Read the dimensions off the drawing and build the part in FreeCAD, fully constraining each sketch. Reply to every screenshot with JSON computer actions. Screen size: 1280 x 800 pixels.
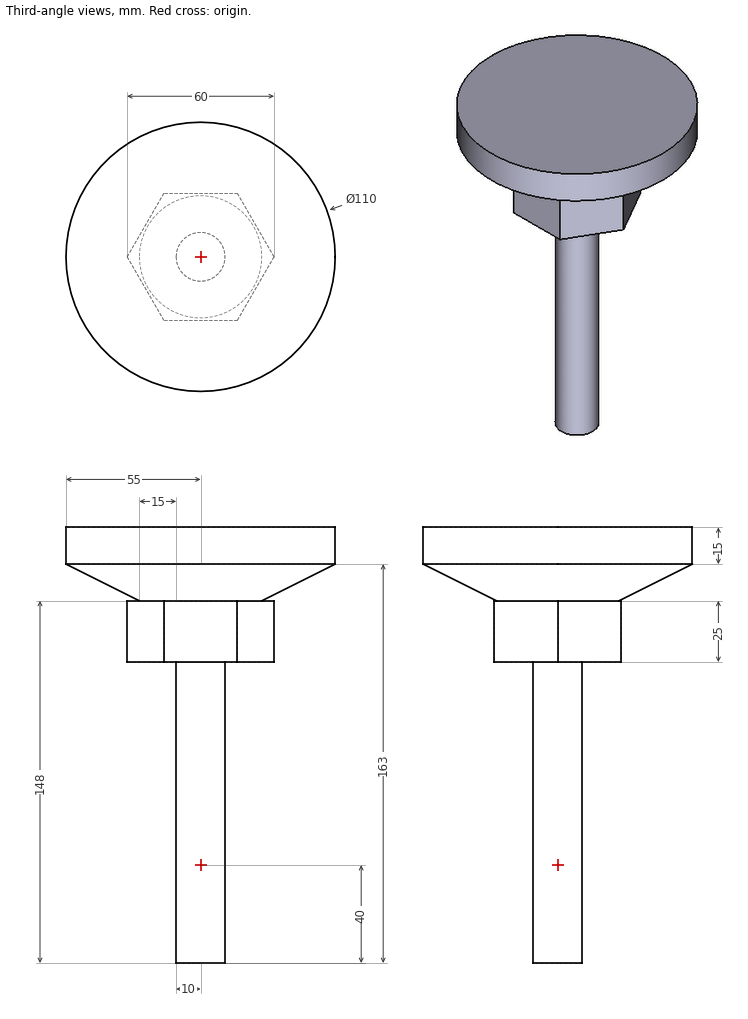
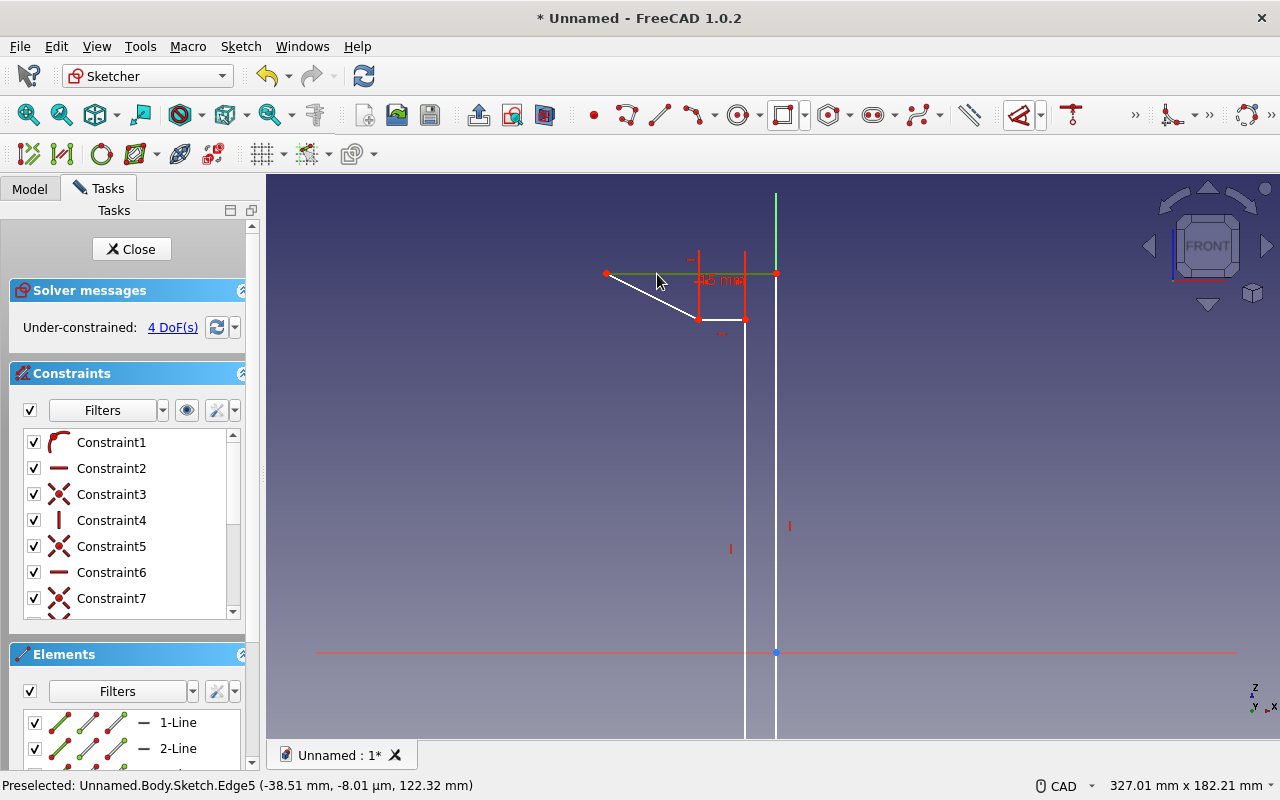
{"action": "left_click", "coordinate": [1040, 116]}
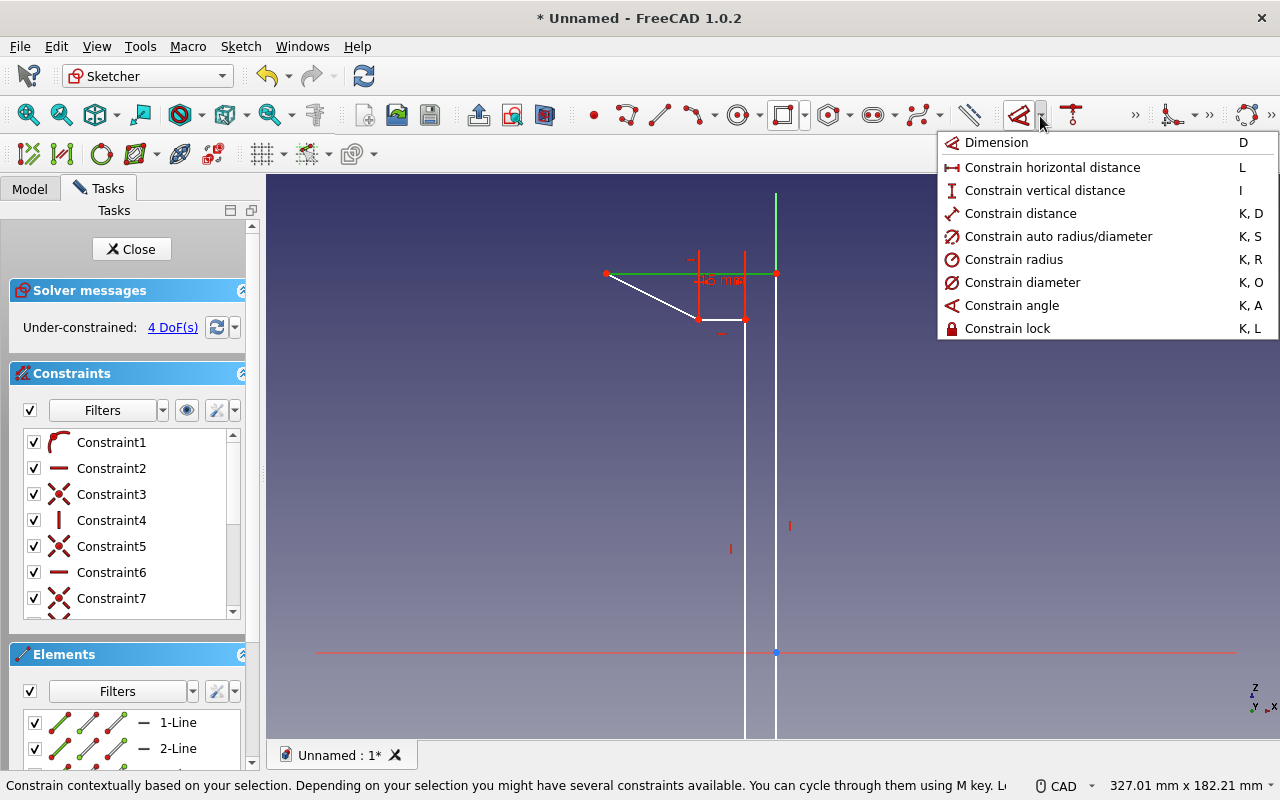
{"action": "left_click", "coordinate": [1108, 168]}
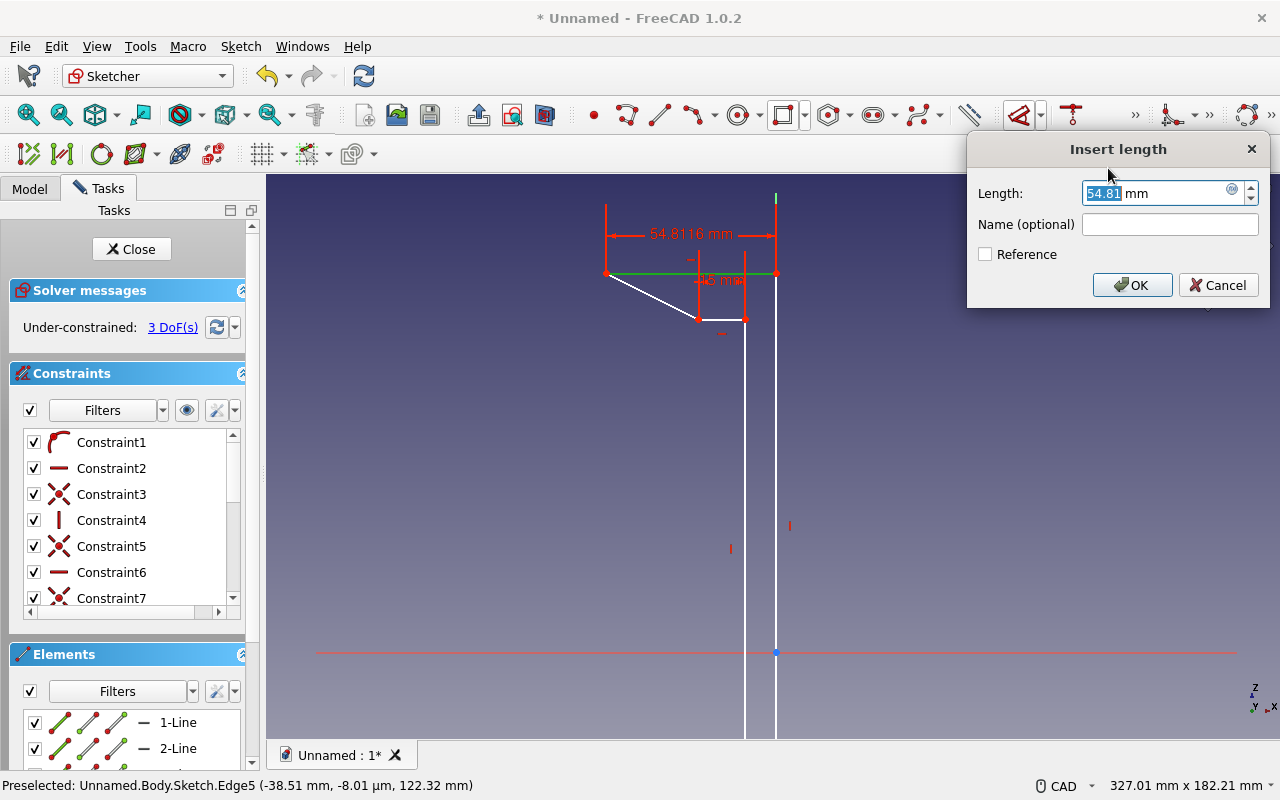
{"action": "type", "text": "55"}
{"action": "key", "text": "Return"}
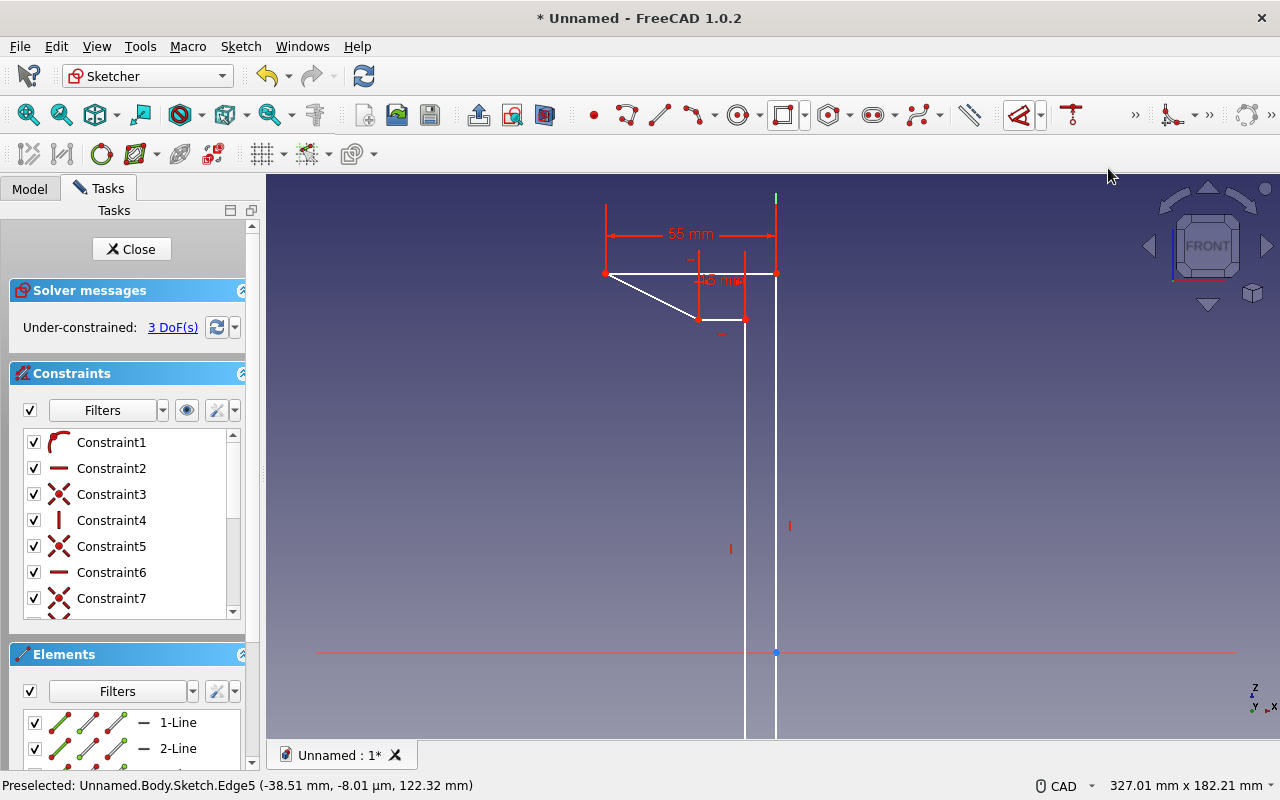
{"action": "left_click", "coordinate": [745, 640]}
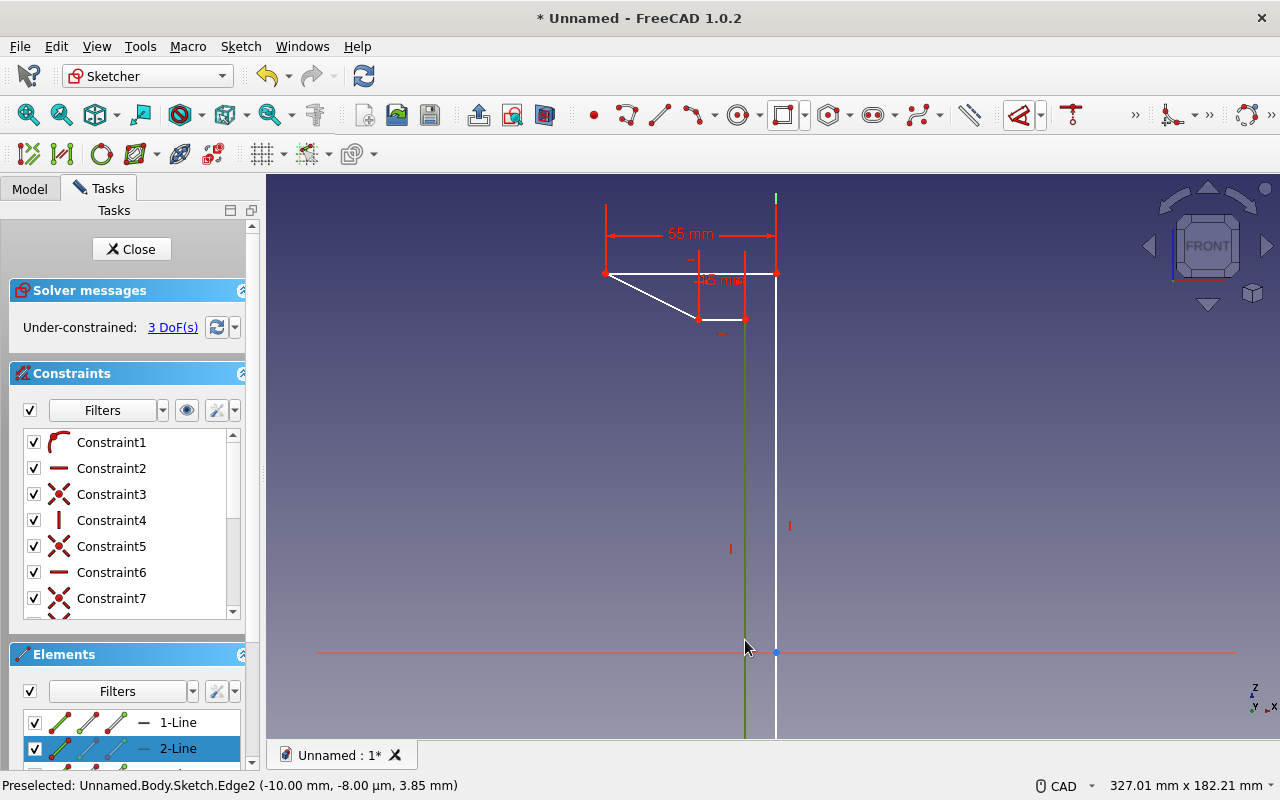
{"action": "left_click", "coordinate": [1040, 116]}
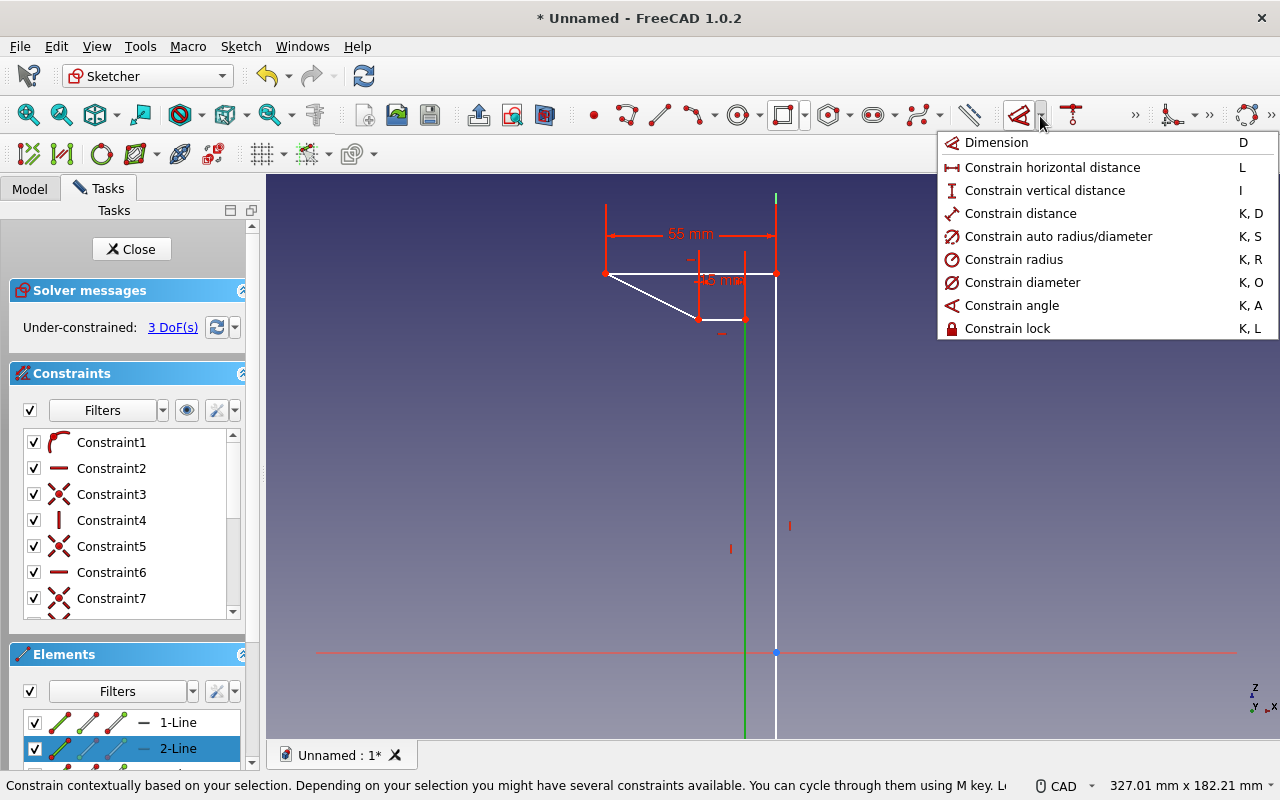
{"action": "left_click", "coordinate": [1108, 190]}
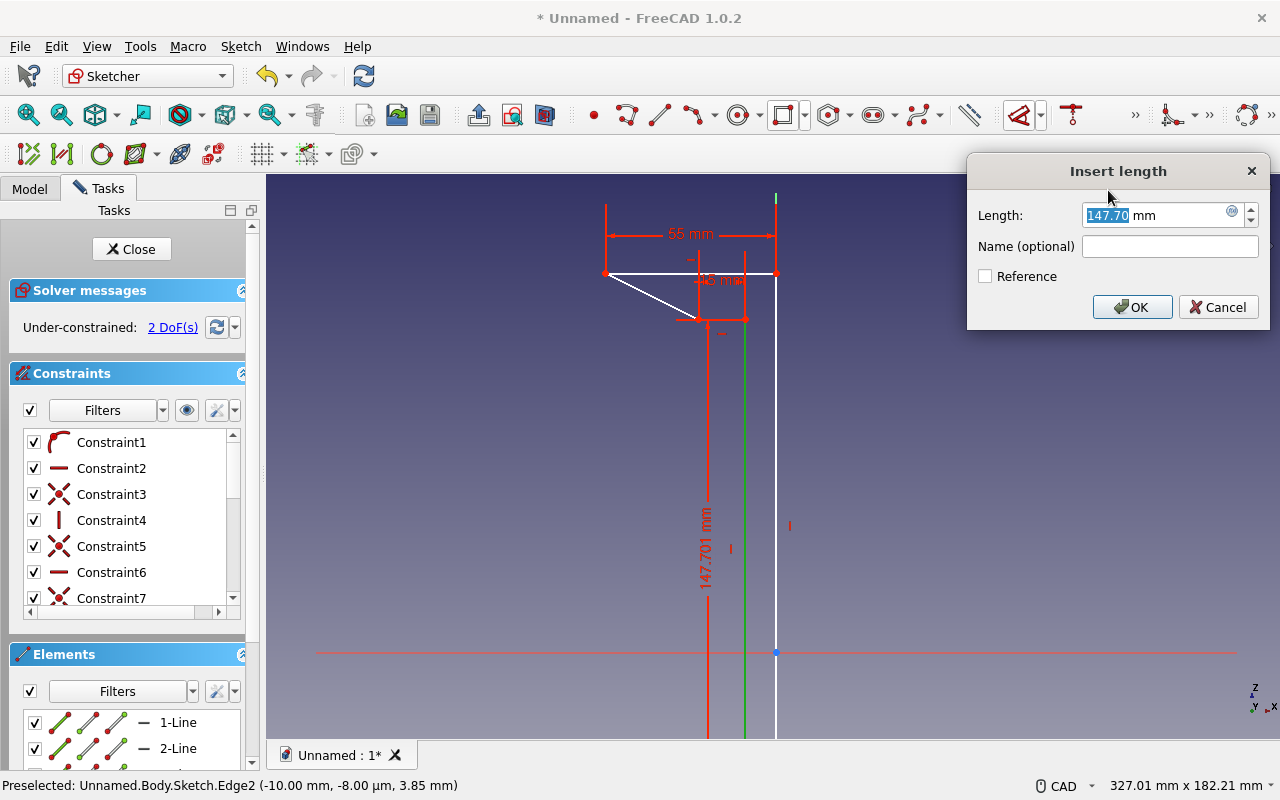
{"action": "type", "text": "148"}
{"action": "key", "text": "Return"}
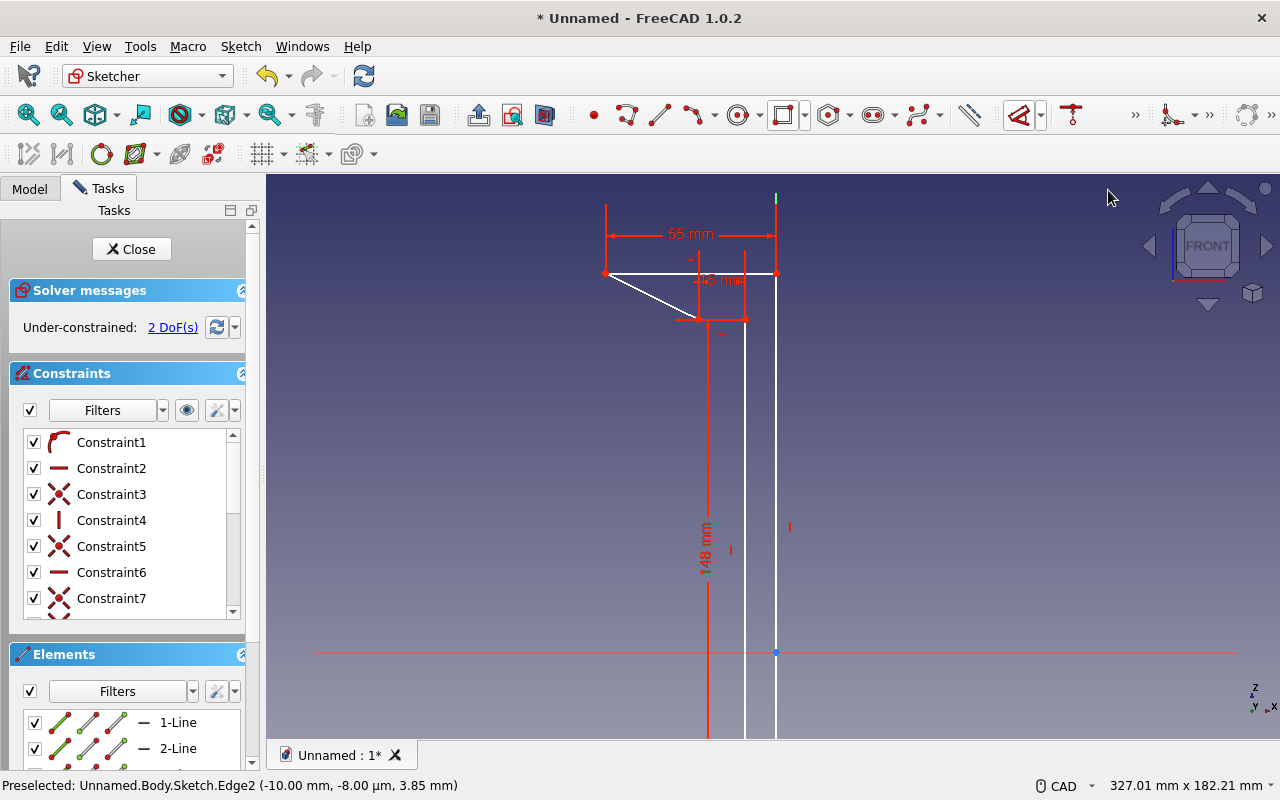
{"action": "left_click", "coordinate": [776, 425]}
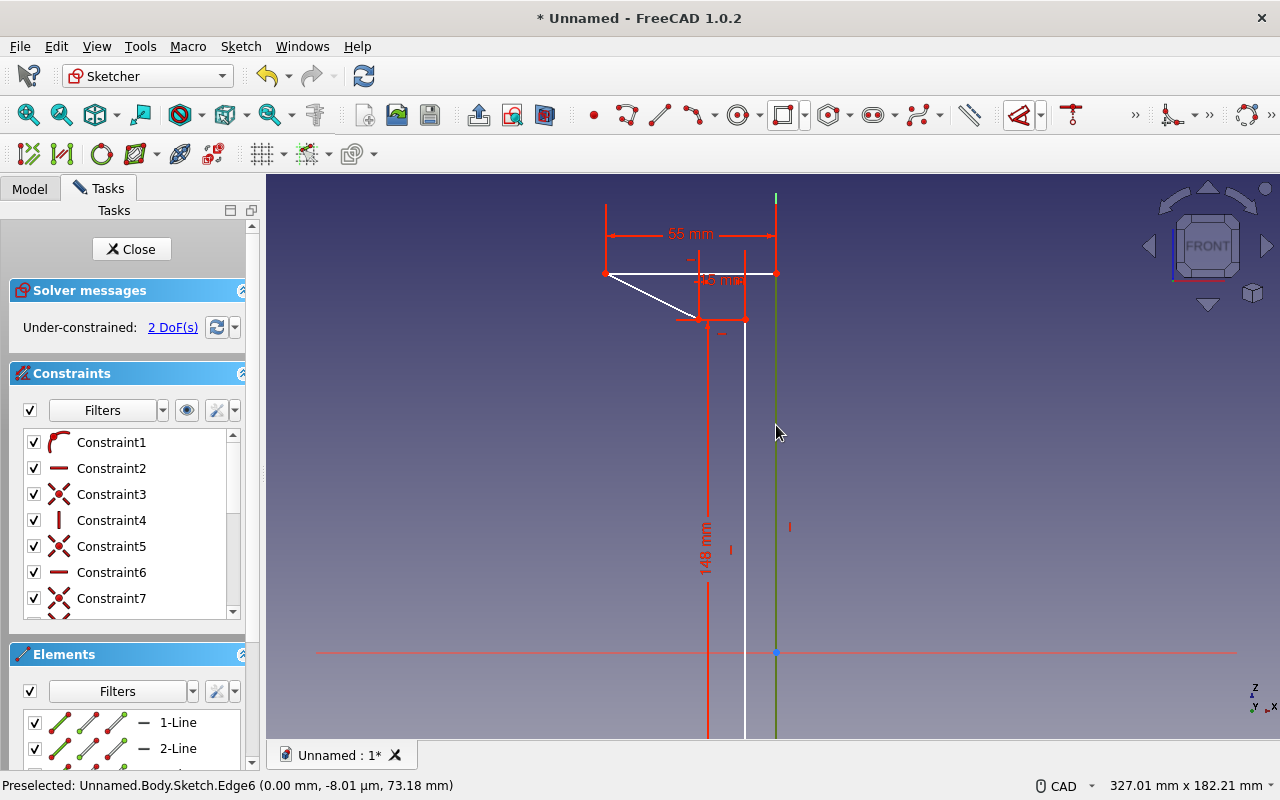
{"action": "key", "text": "i"}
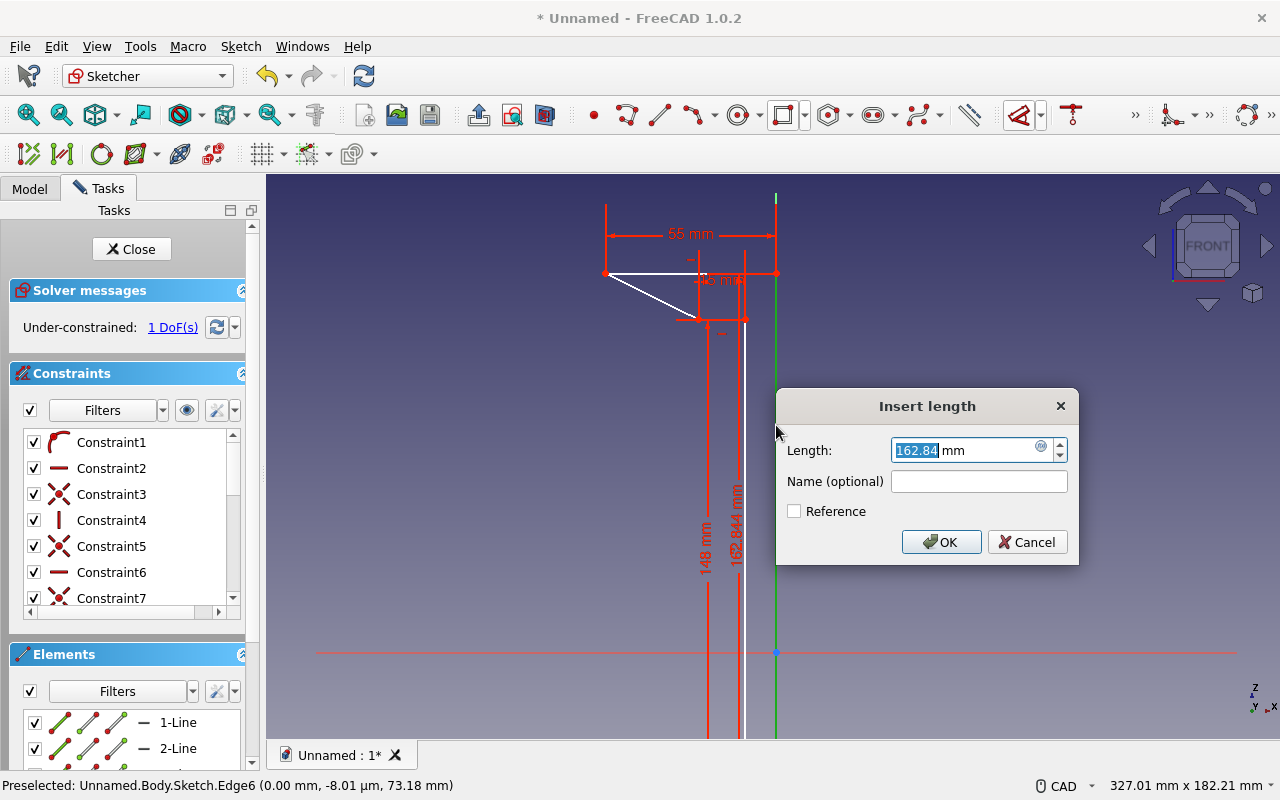
{"action": "type", "text": "163"}
{"action": "key", "text": "Return"}